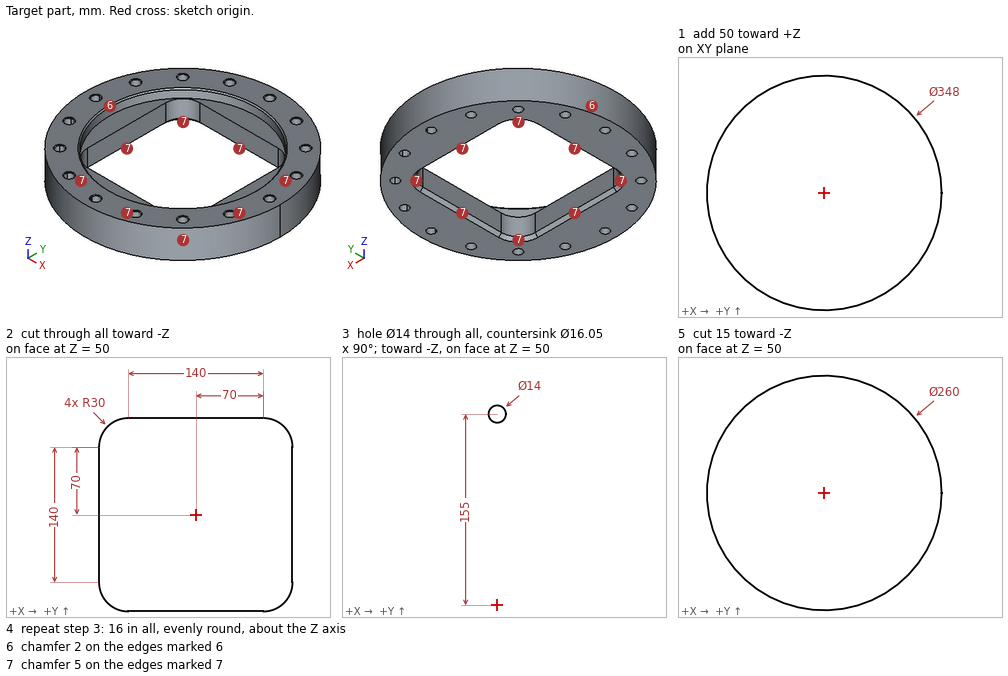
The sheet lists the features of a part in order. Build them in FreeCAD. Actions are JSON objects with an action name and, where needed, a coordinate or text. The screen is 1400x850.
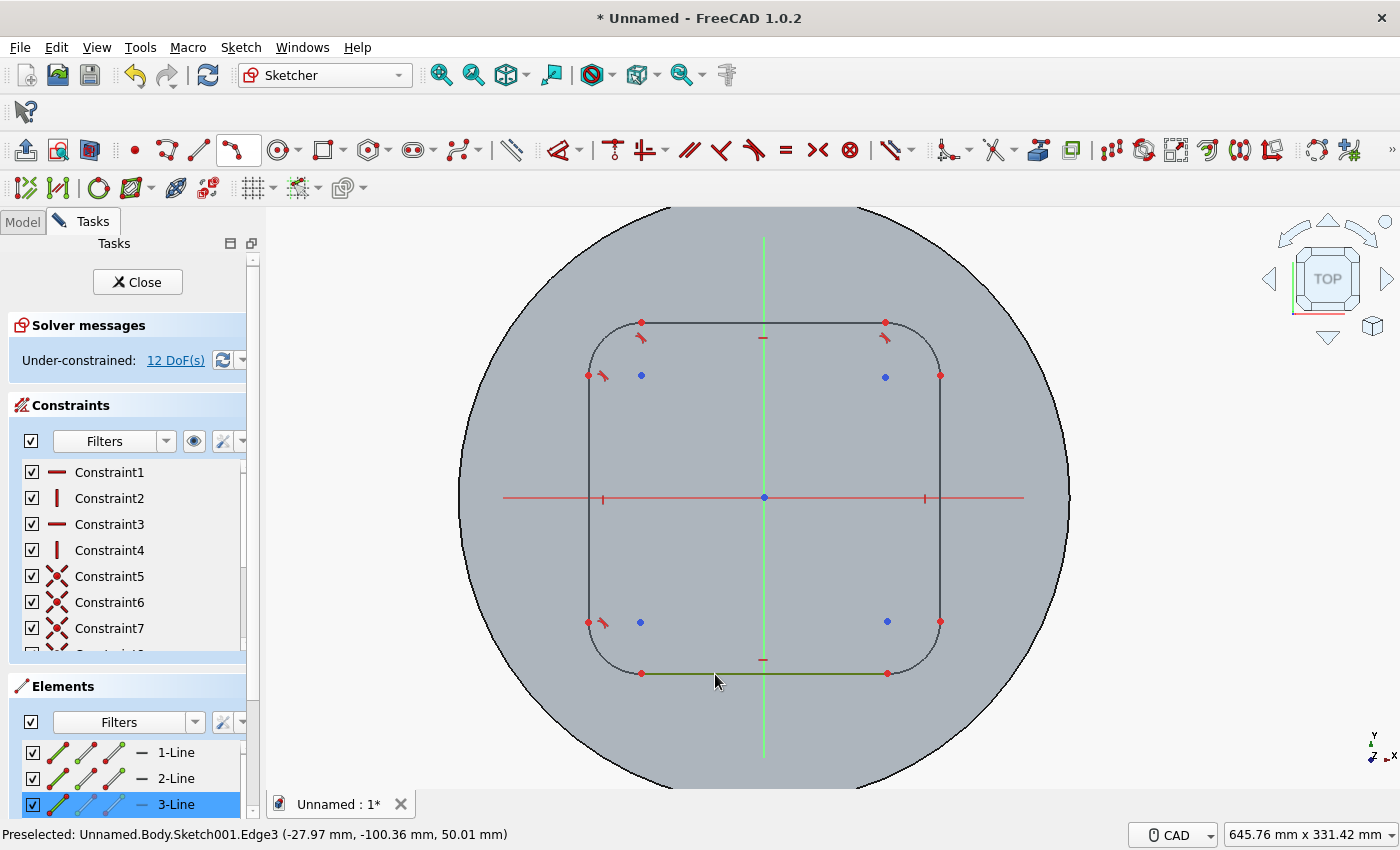
{"action": "left_click", "coordinate": [595, 646]}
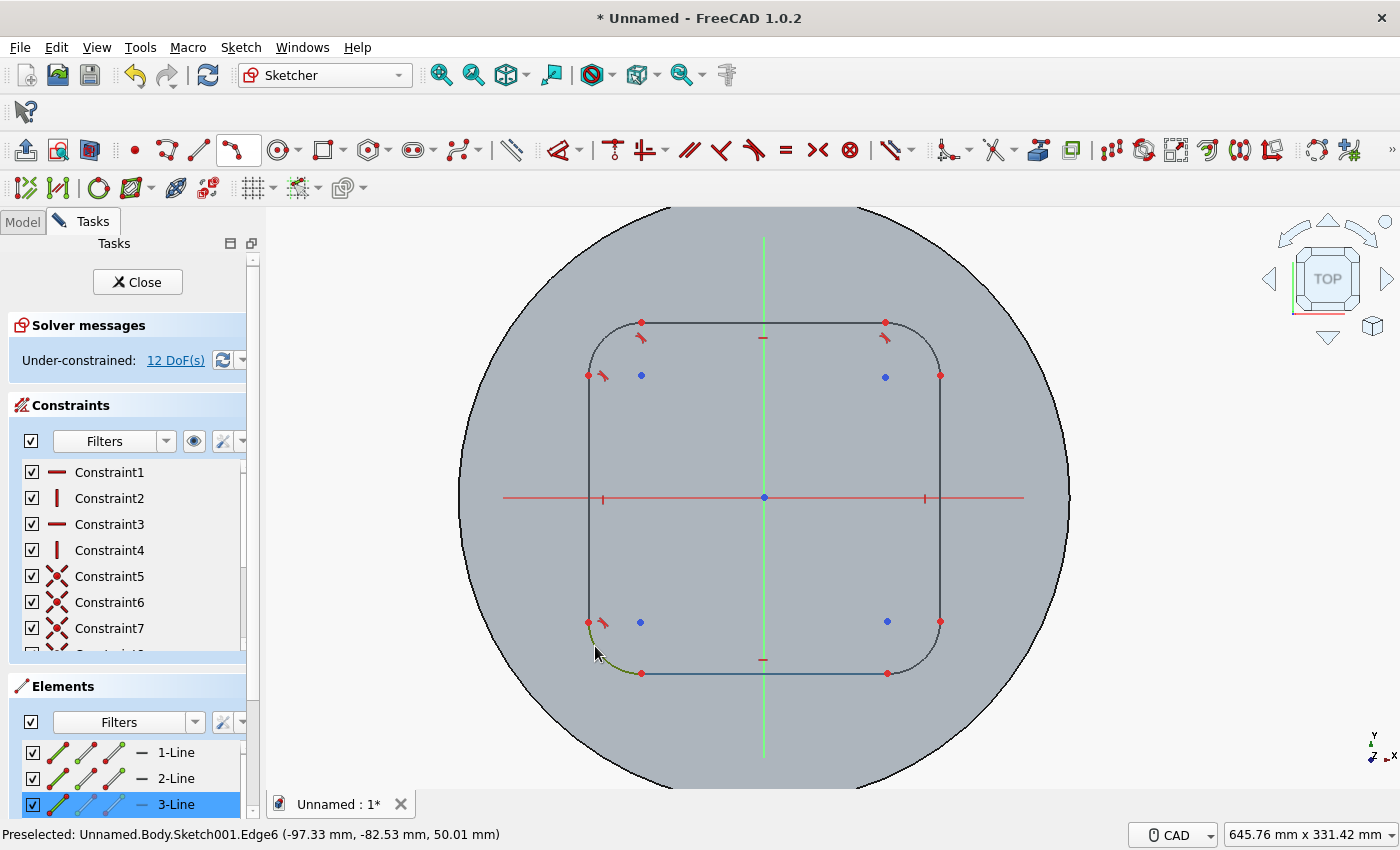
{"action": "left_click", "coordinate": [754, 150]}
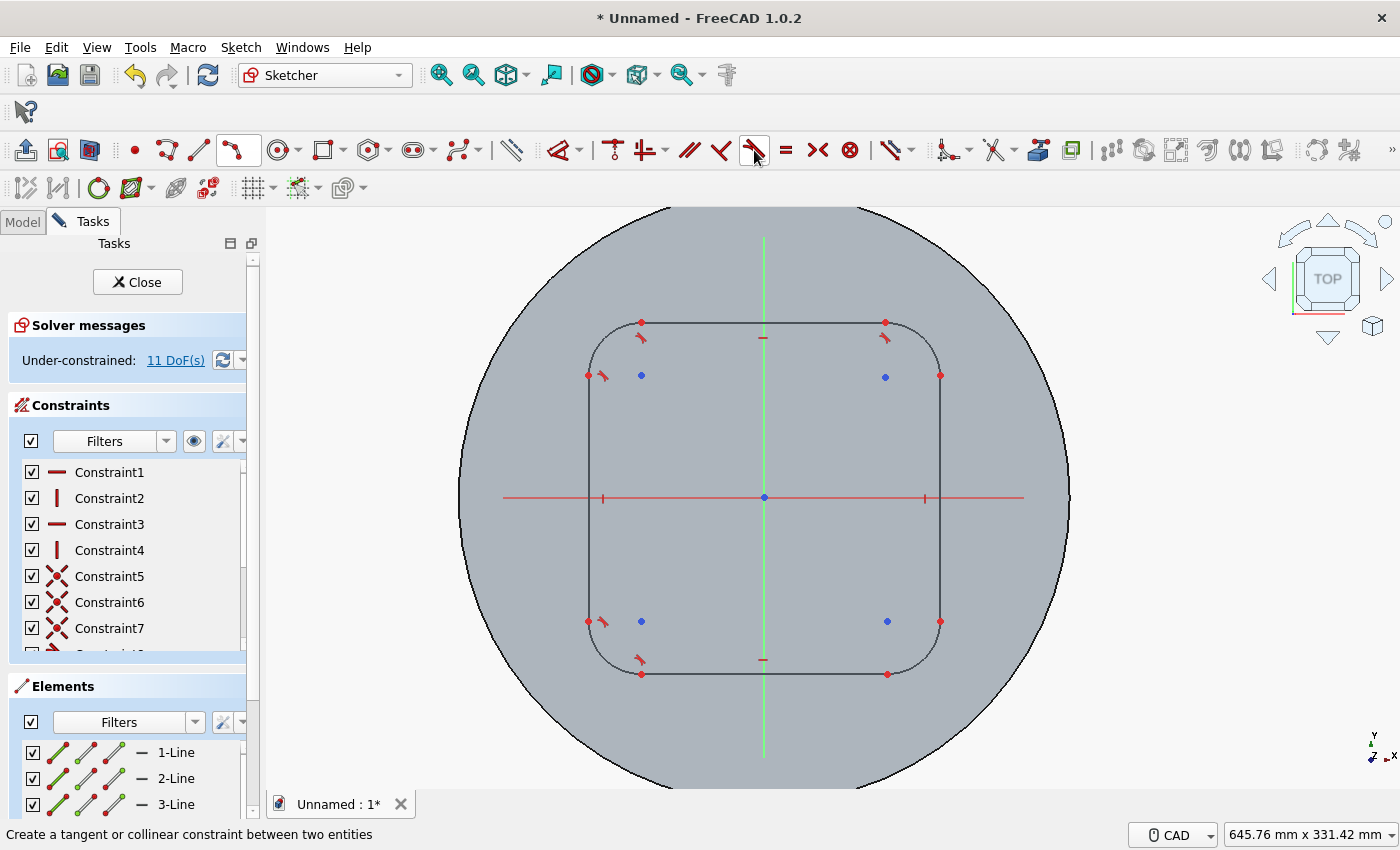
{"action": "left_click", "coordinate": [715, 674]}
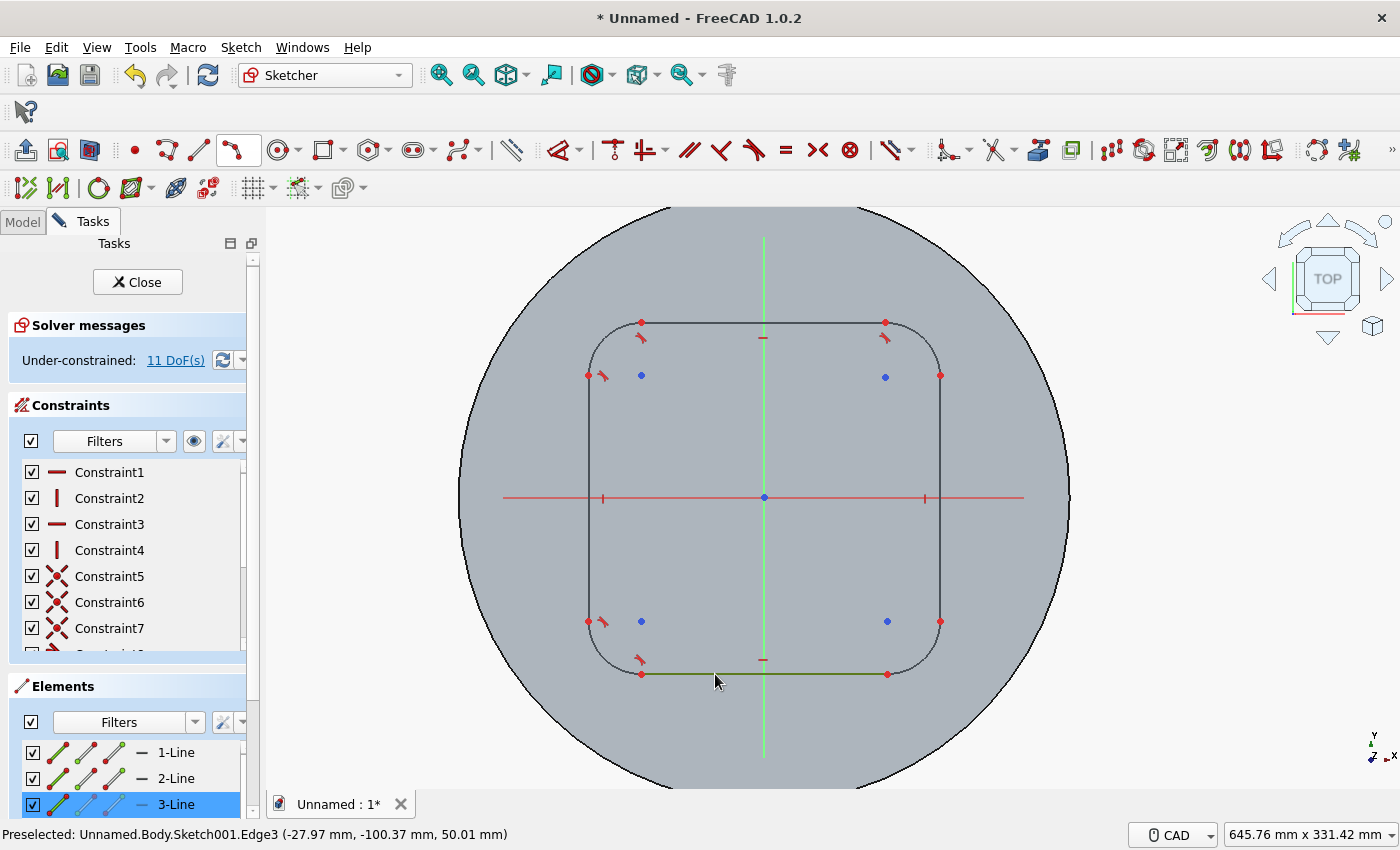
{"action": "left_click", "coordinate": [911, 668]}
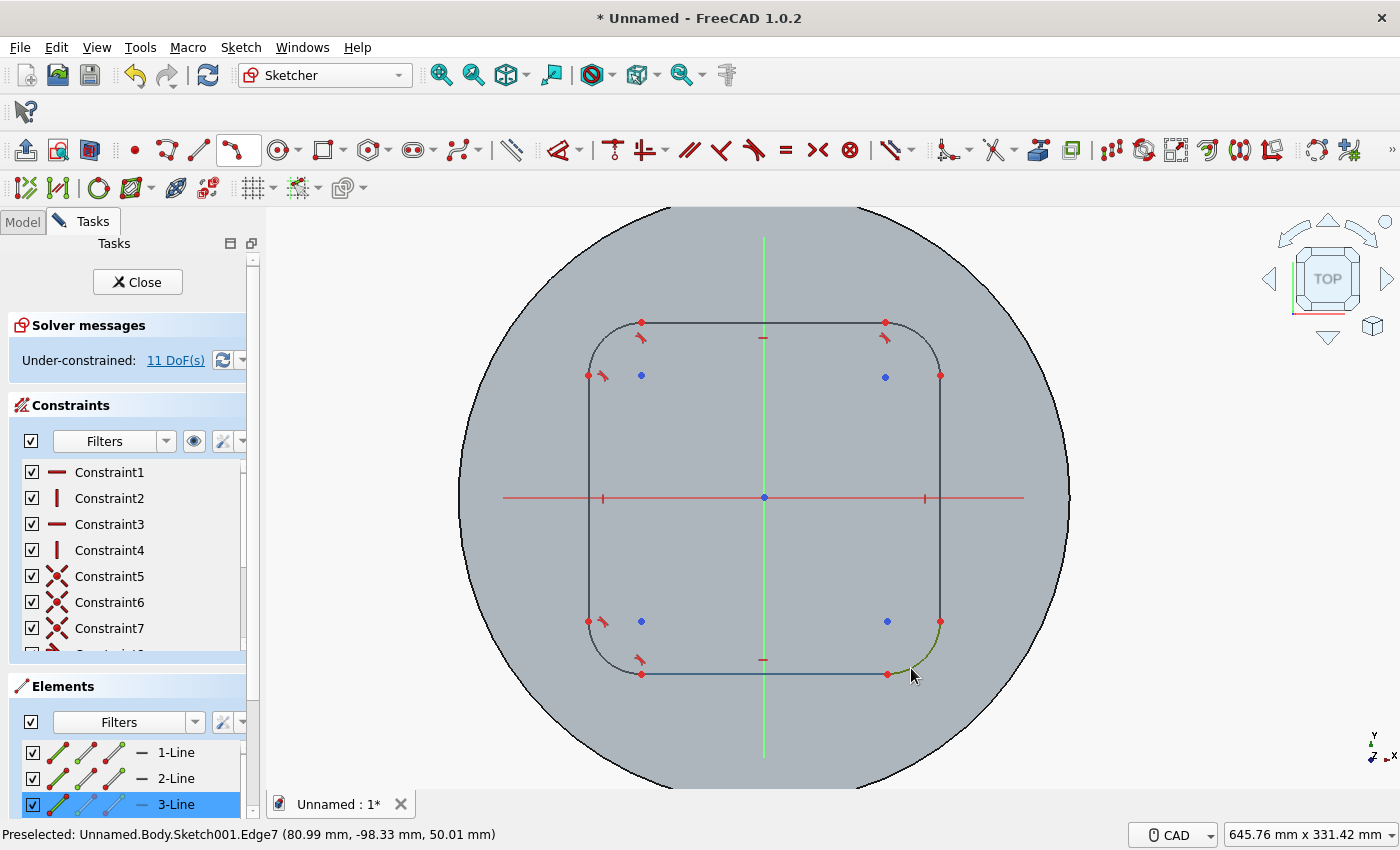
{"action": "left_click", "coordinate": [754, 150]}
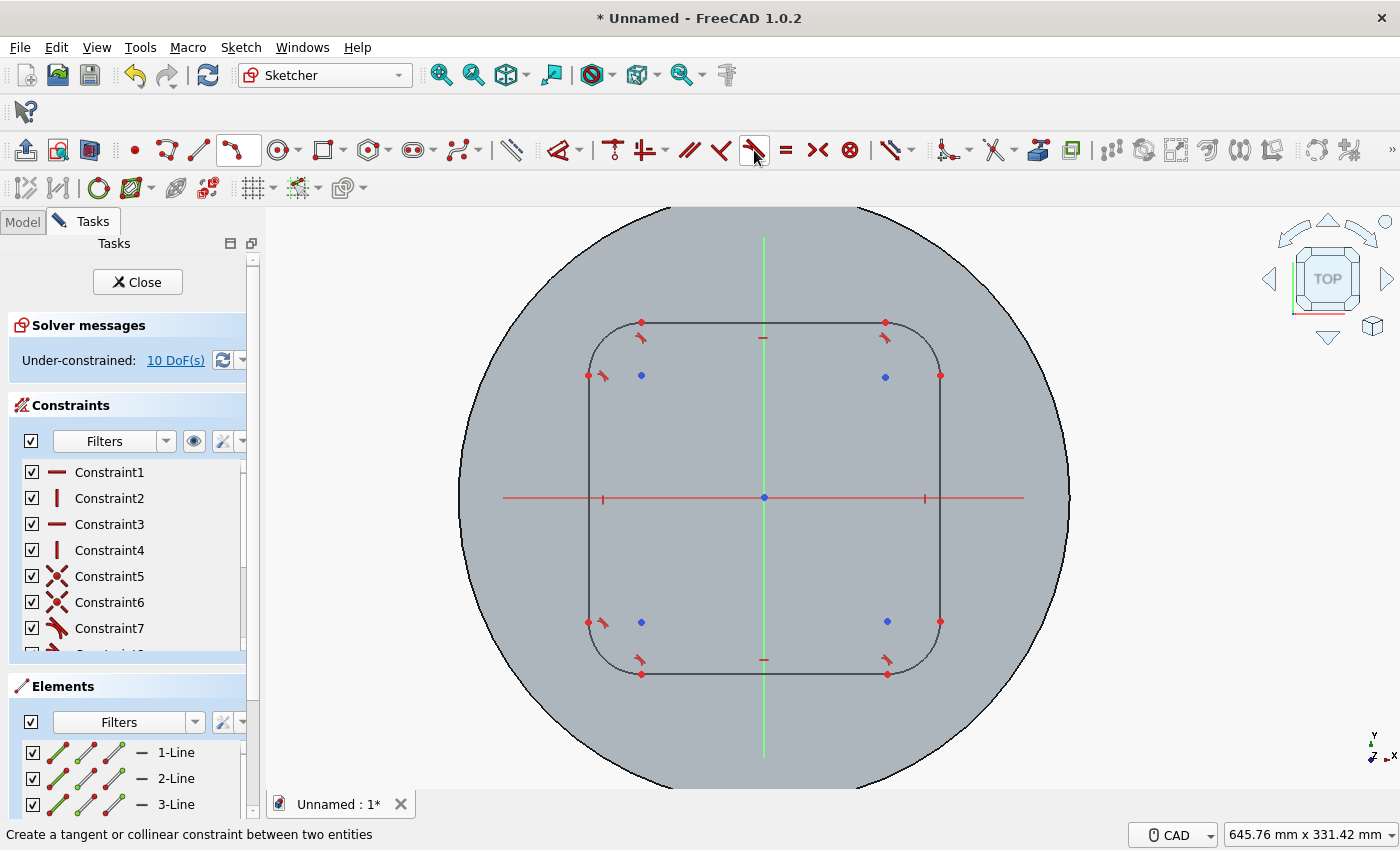
{"action": "left_click", "coordinate": [940, 548]}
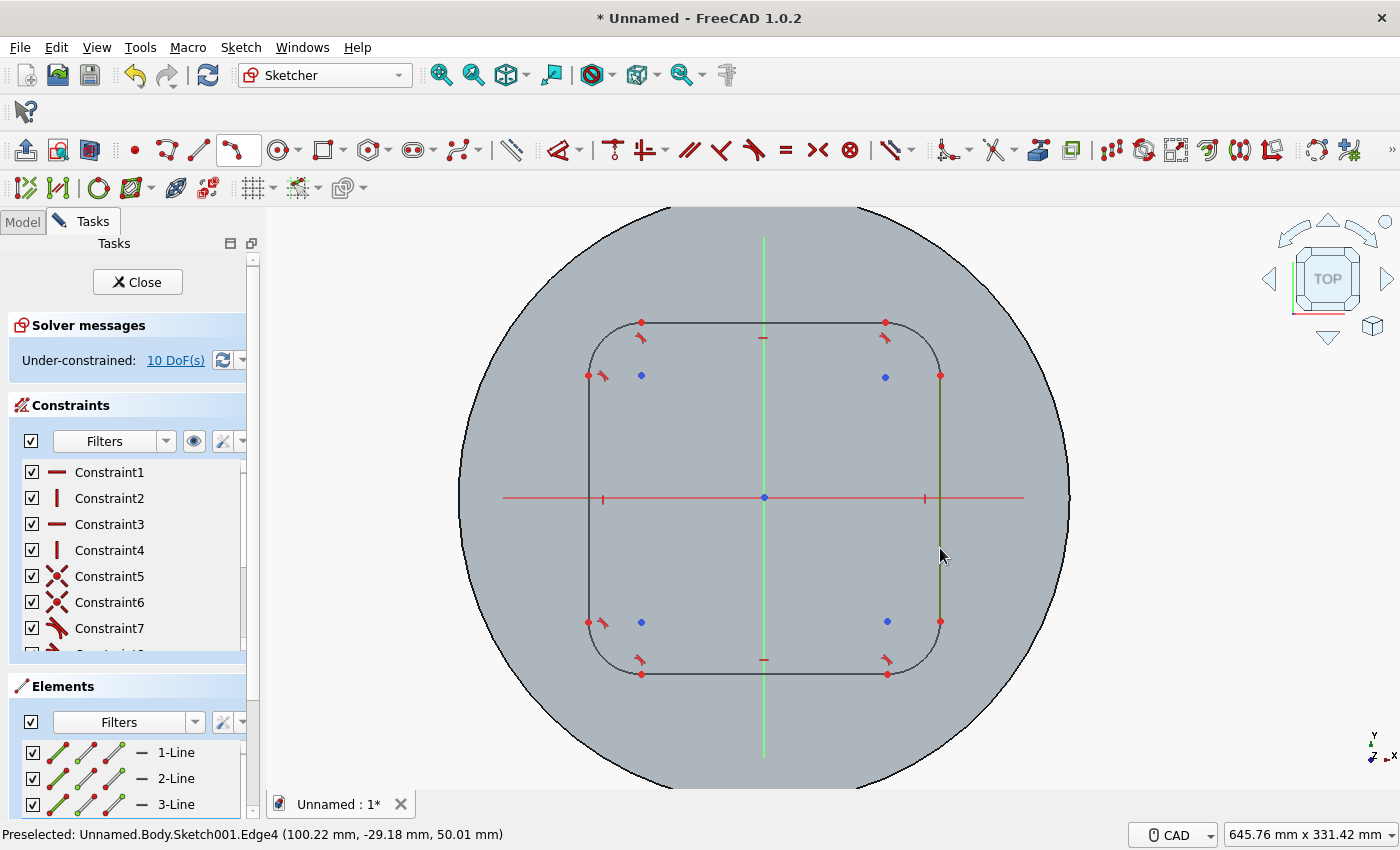
{"action": "left_click", "coordinate": [911, 669]}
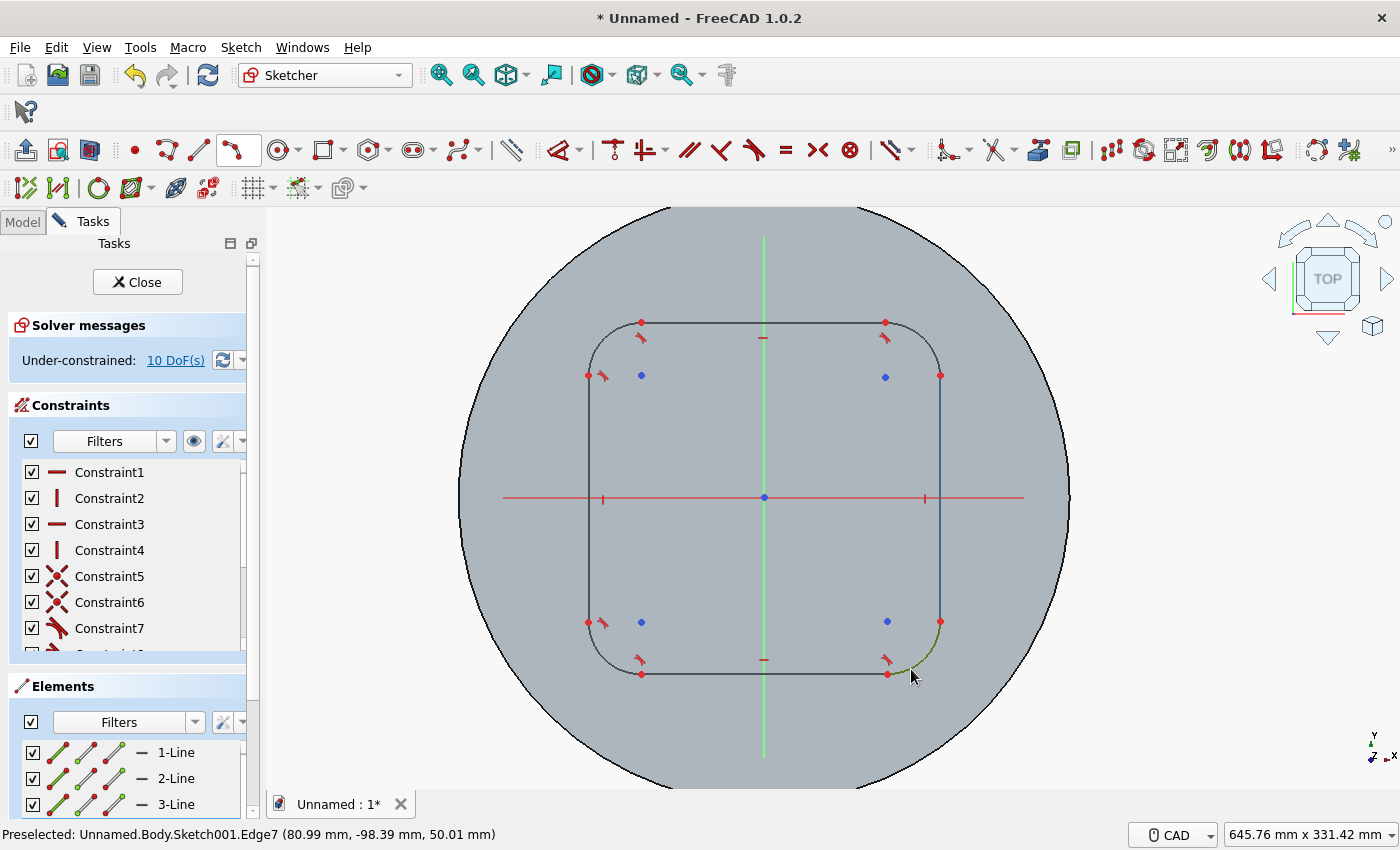
{"action": "left_click", "coordinate": [754, 150]}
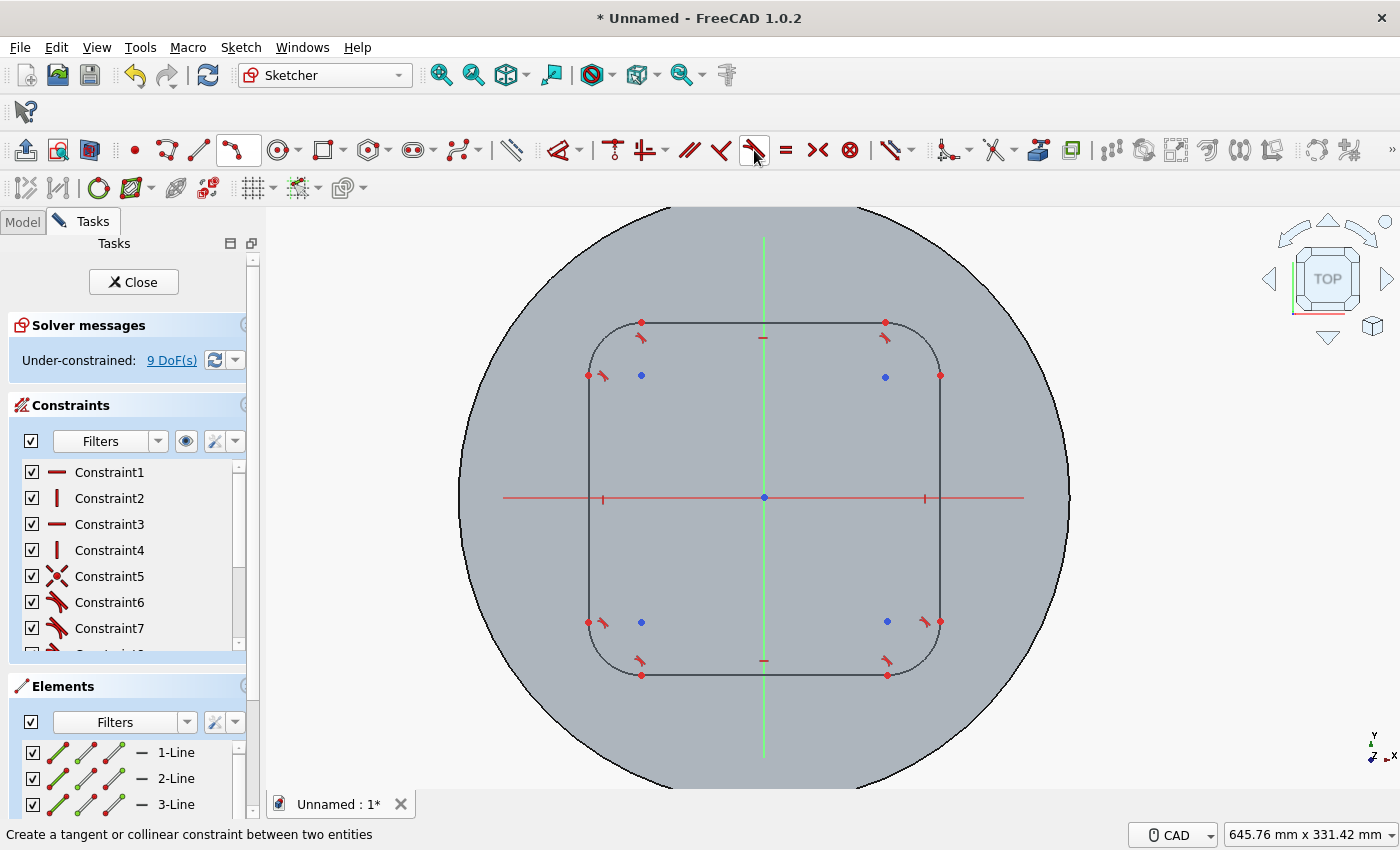
{"action": "left_click", "coordinate": [940, 548]}